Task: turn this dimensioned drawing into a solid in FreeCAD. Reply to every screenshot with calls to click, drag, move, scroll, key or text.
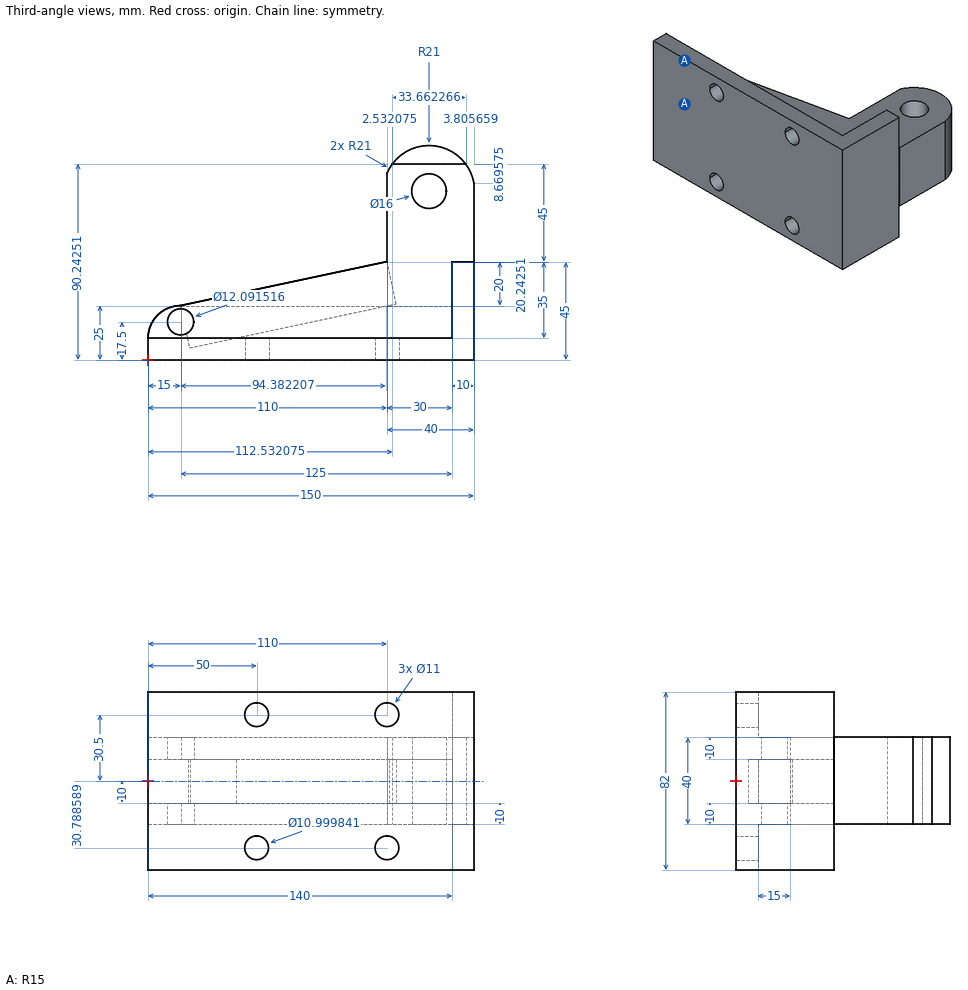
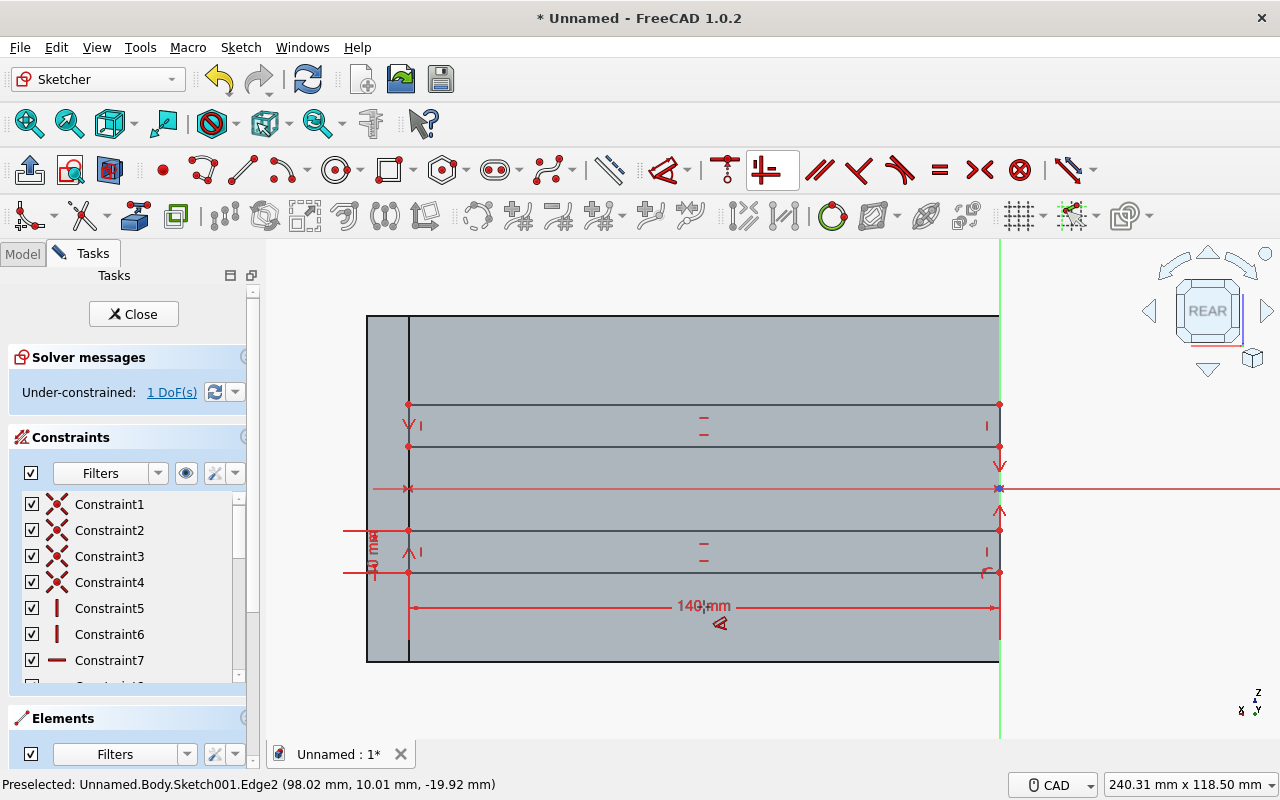
click(409, 531)
click(1034, 510)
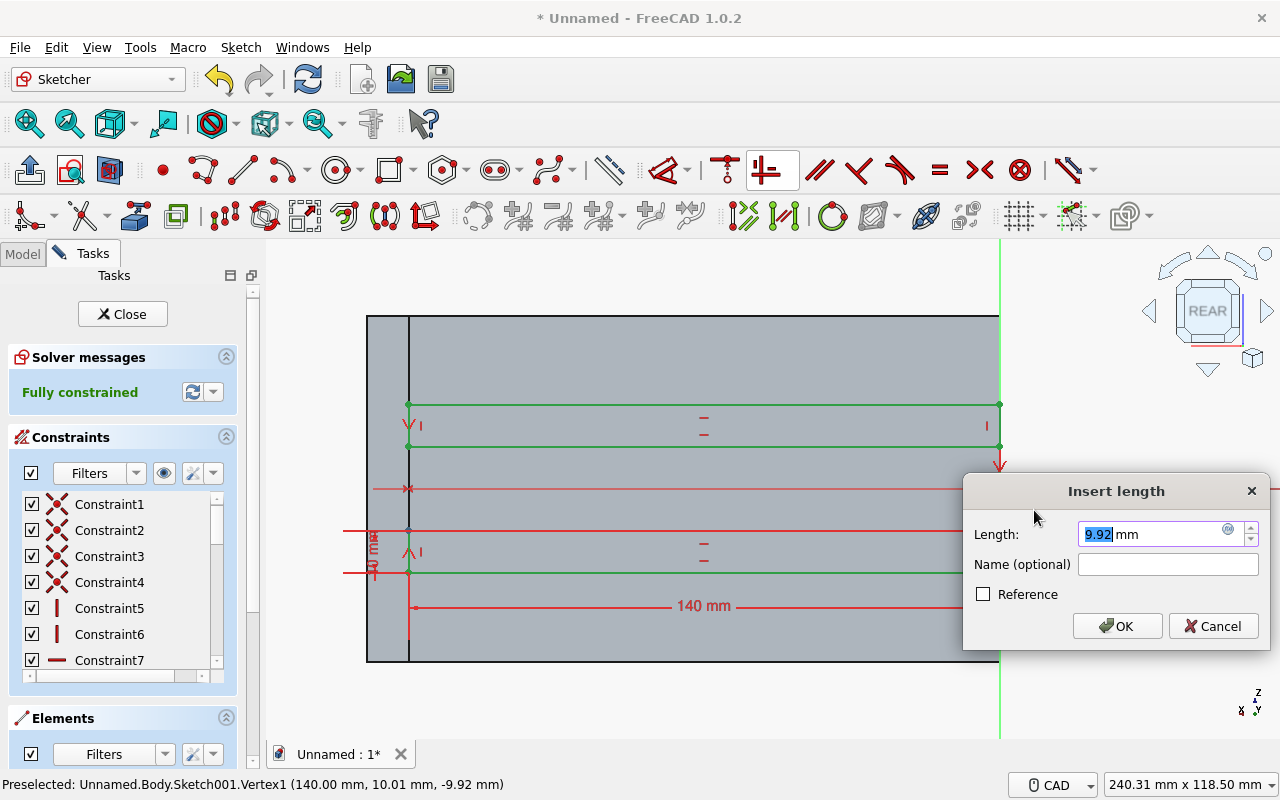
text(10)
key(Return)
key(Escape)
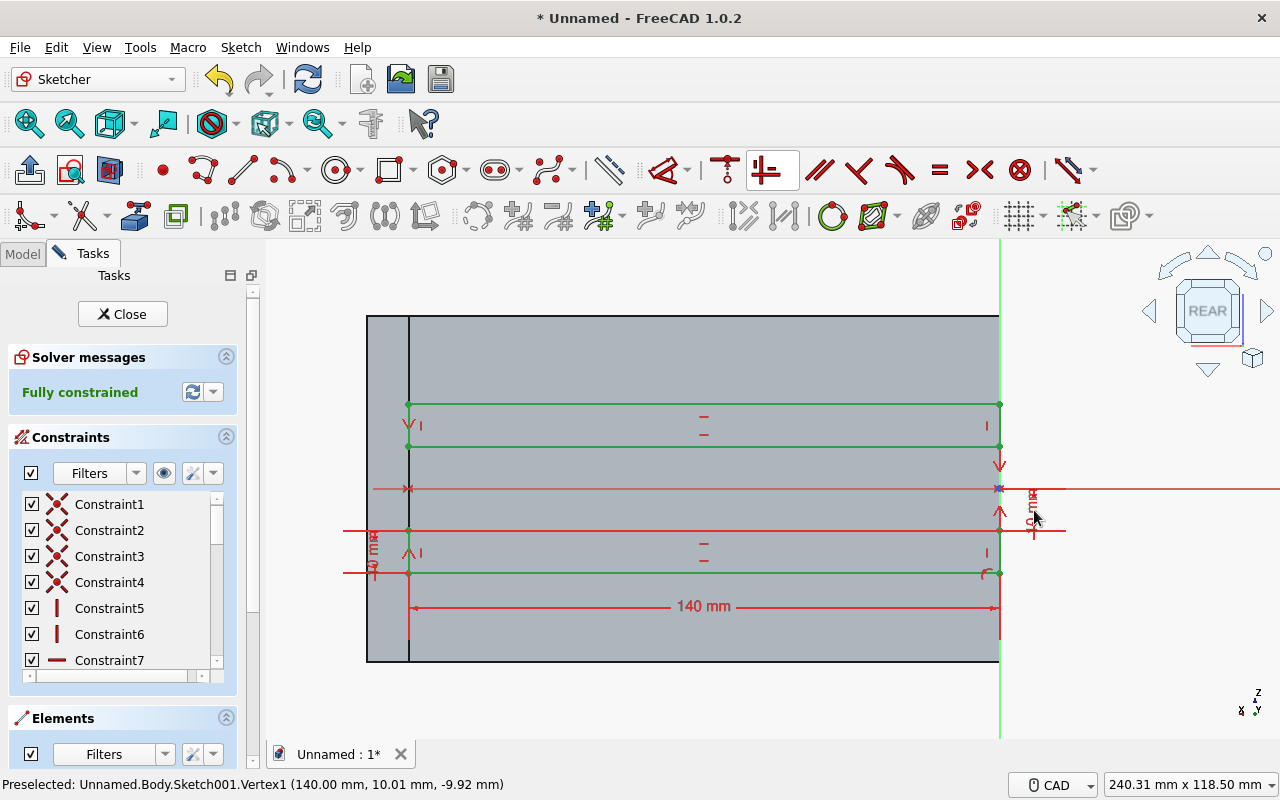
click(123, 314)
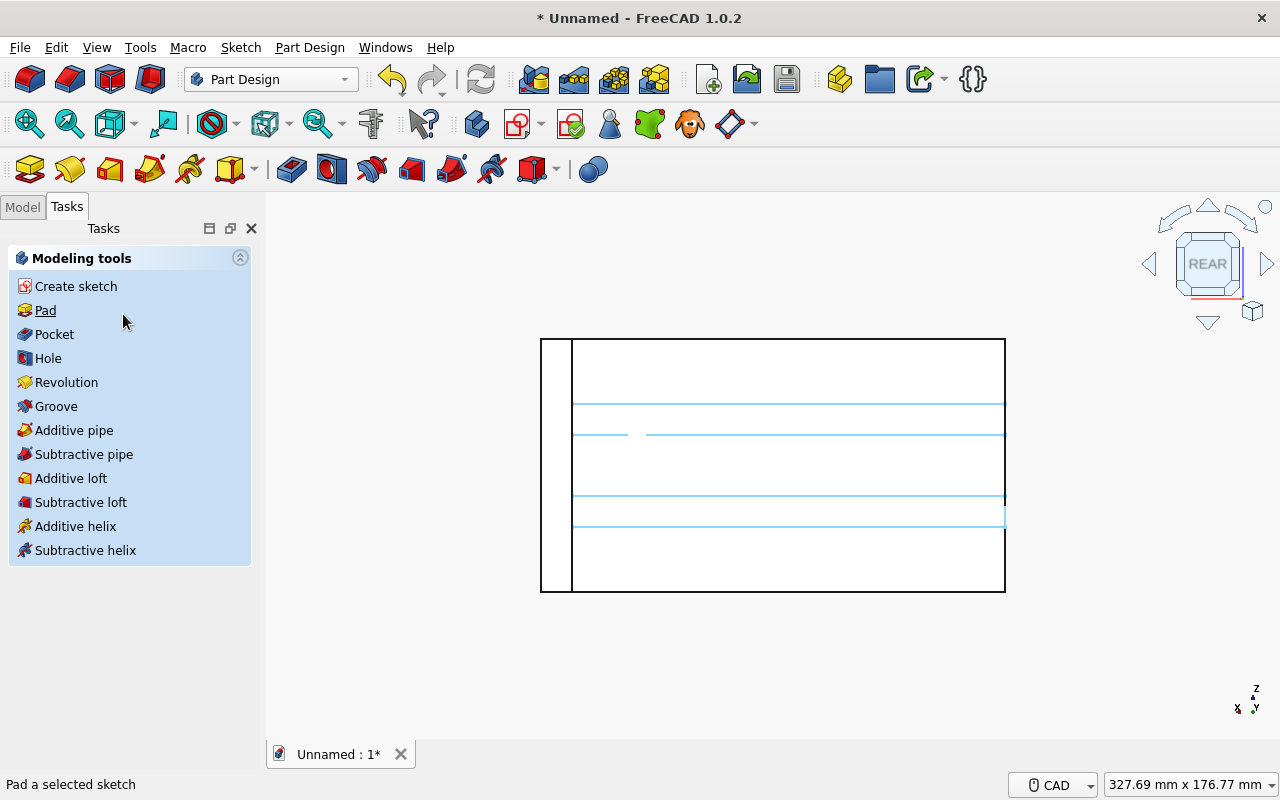
click(30, 170)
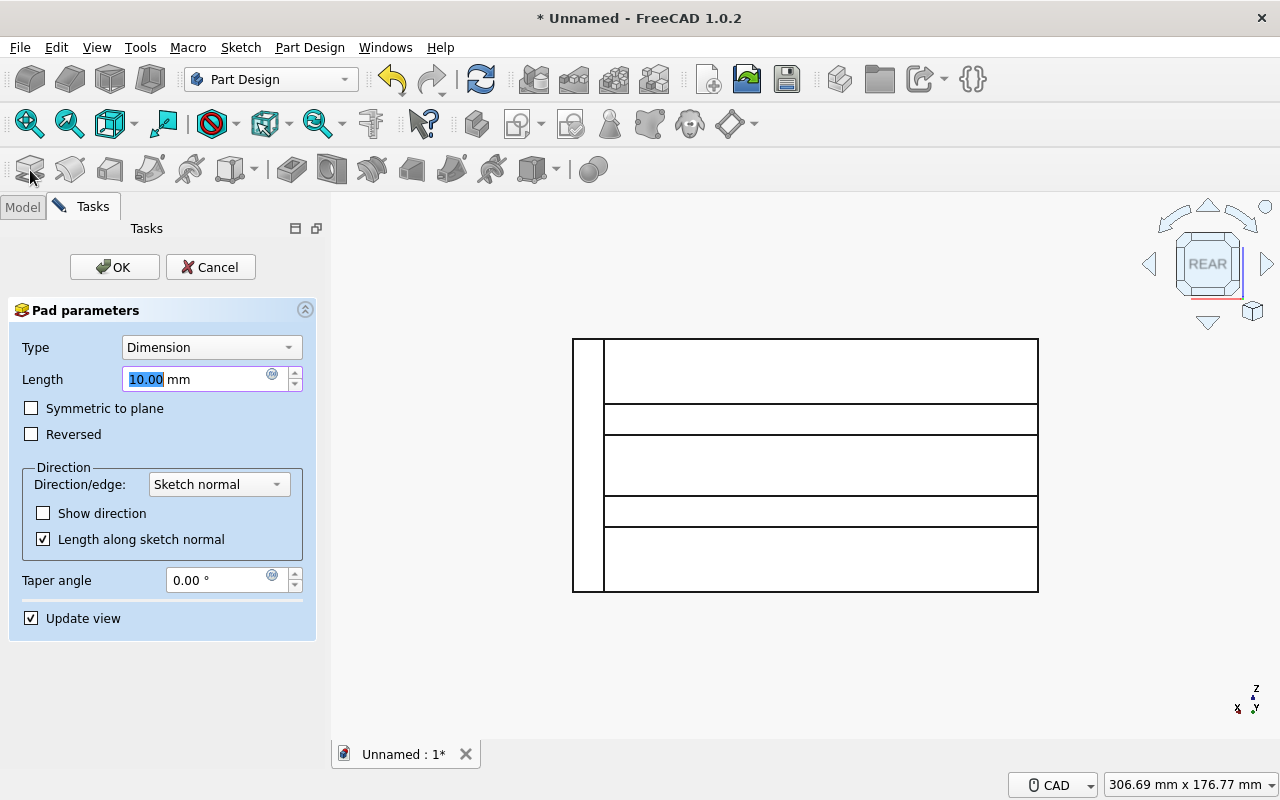
text(15)
key(Tab)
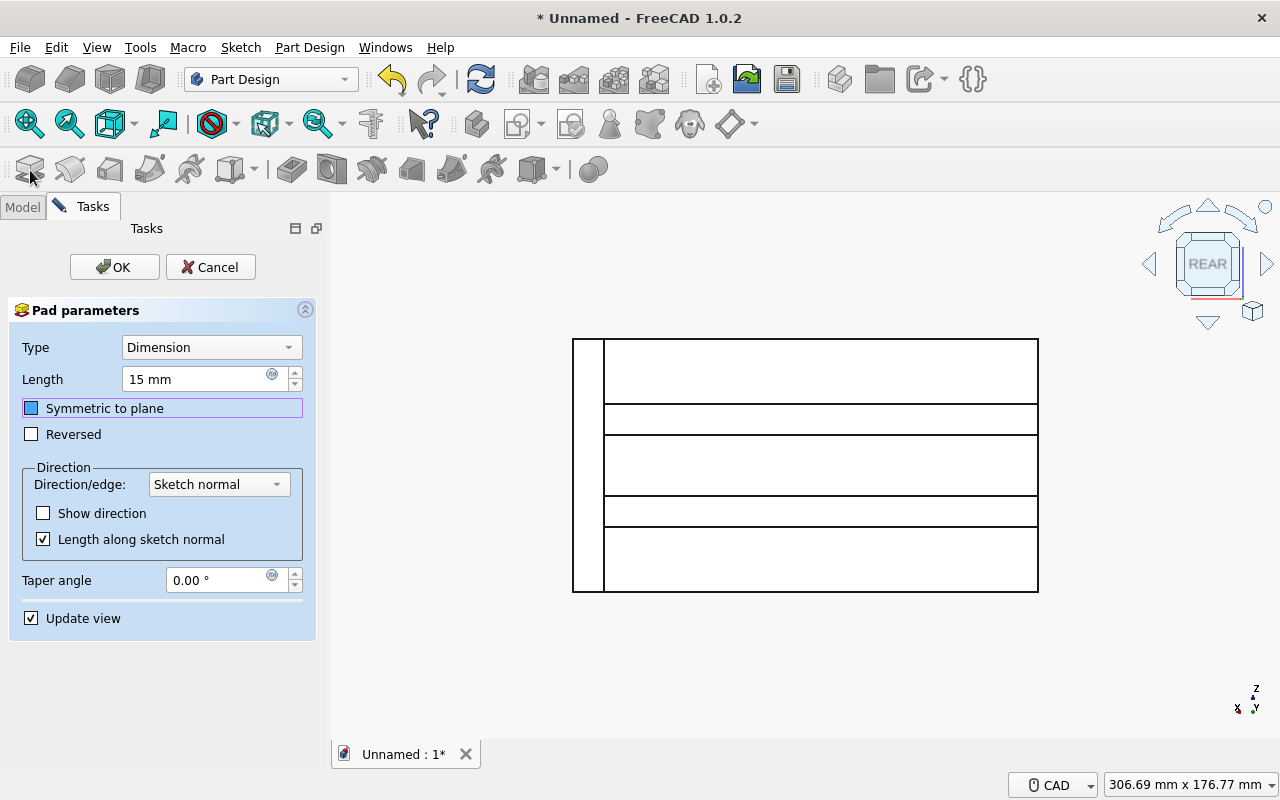
click(115, 267)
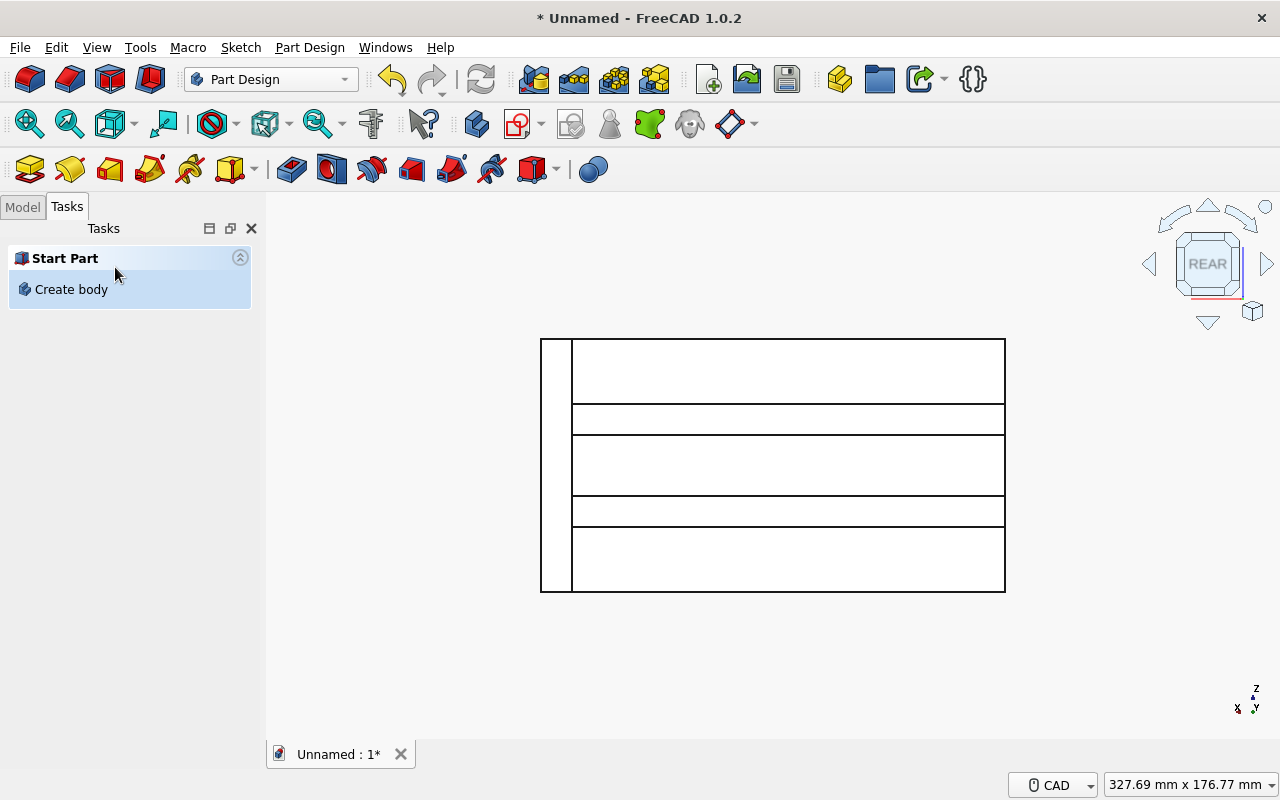
click(1005, 511)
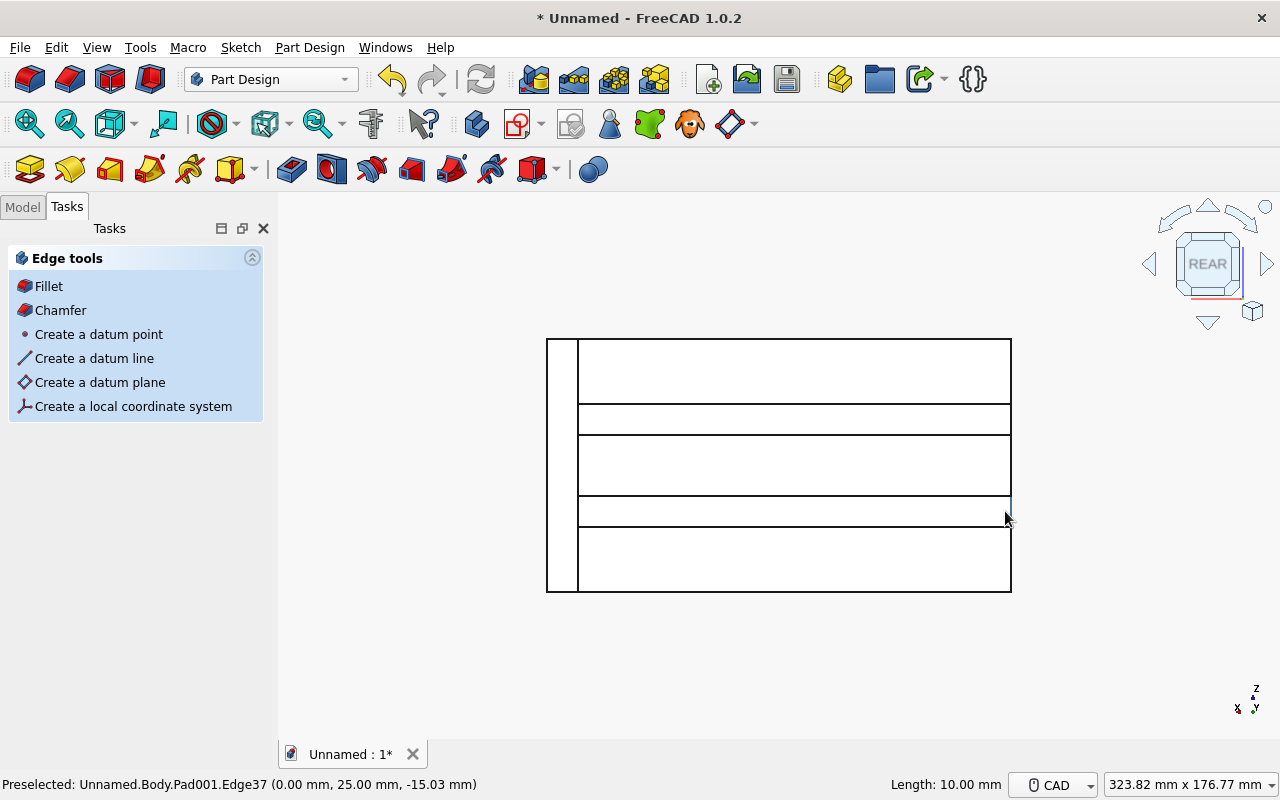
click(1011, 418, ctrl)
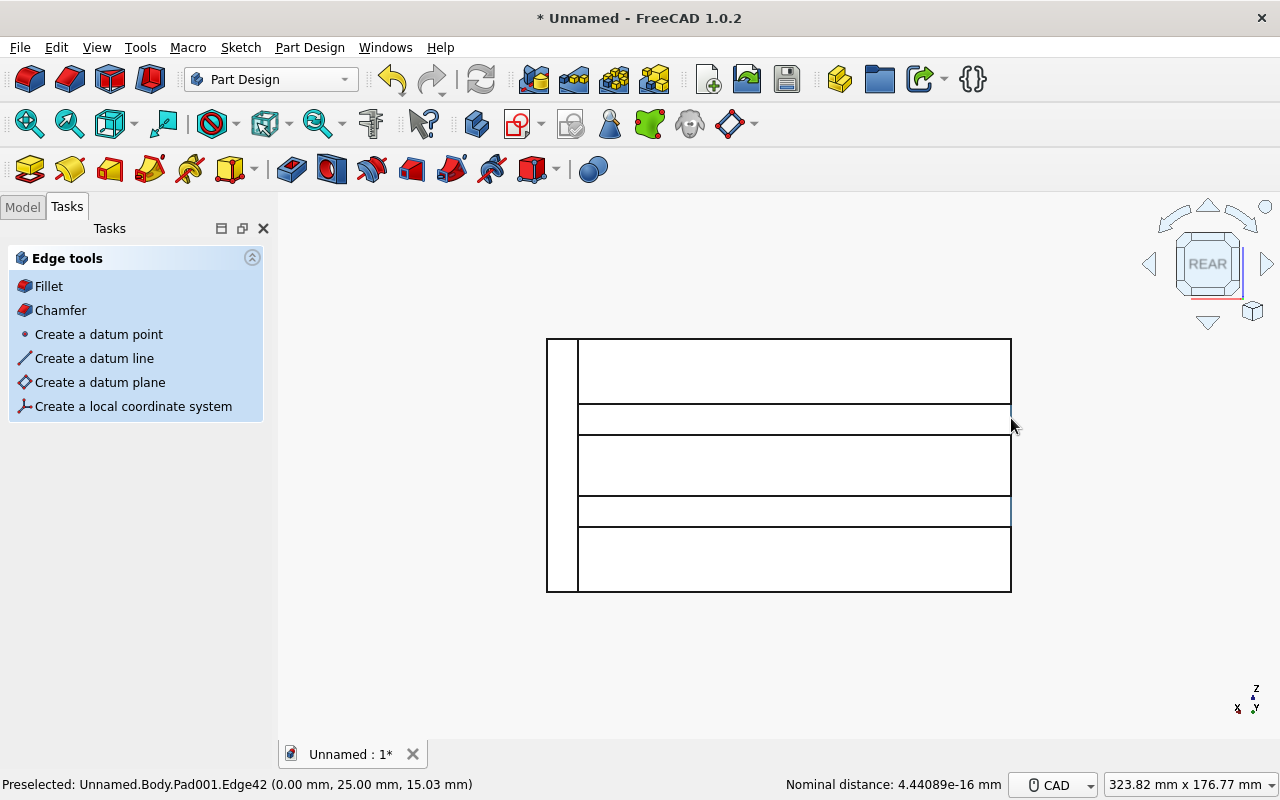
click(30, 80)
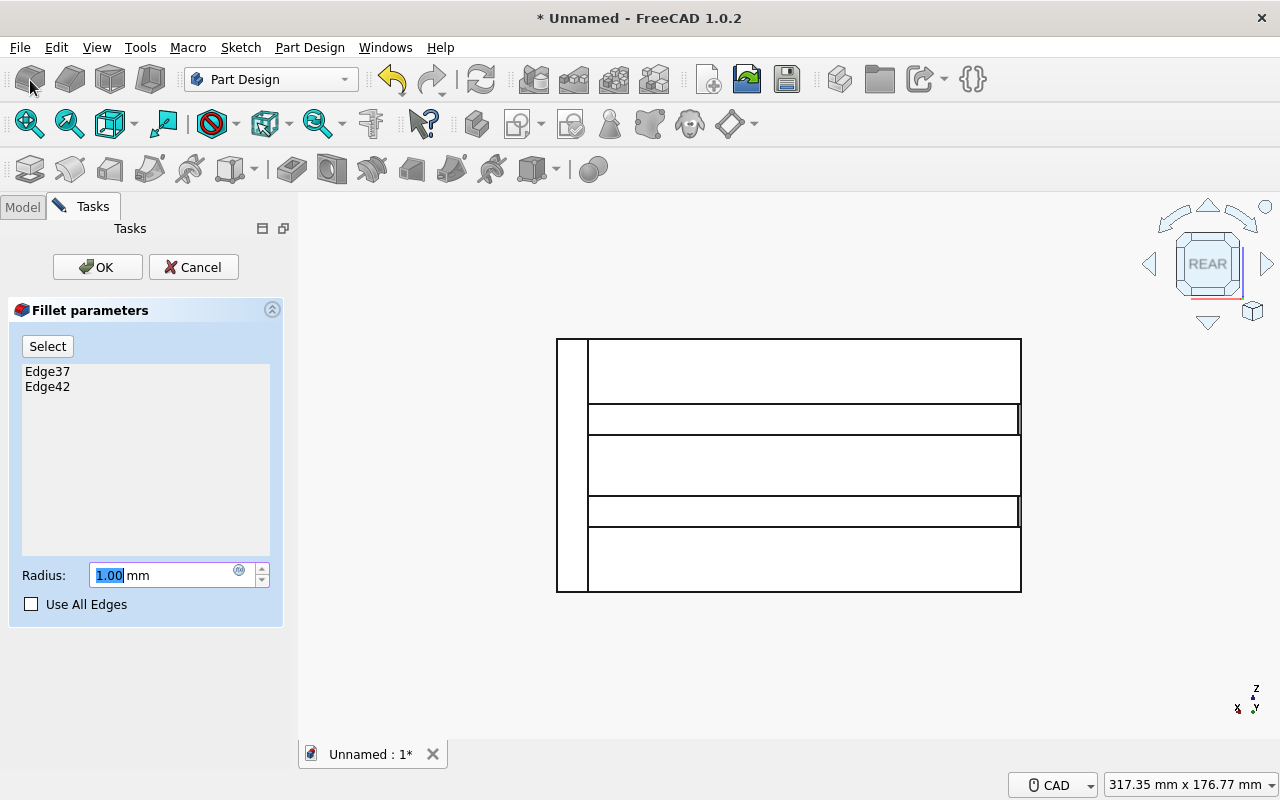
text(15)
key(Tab)